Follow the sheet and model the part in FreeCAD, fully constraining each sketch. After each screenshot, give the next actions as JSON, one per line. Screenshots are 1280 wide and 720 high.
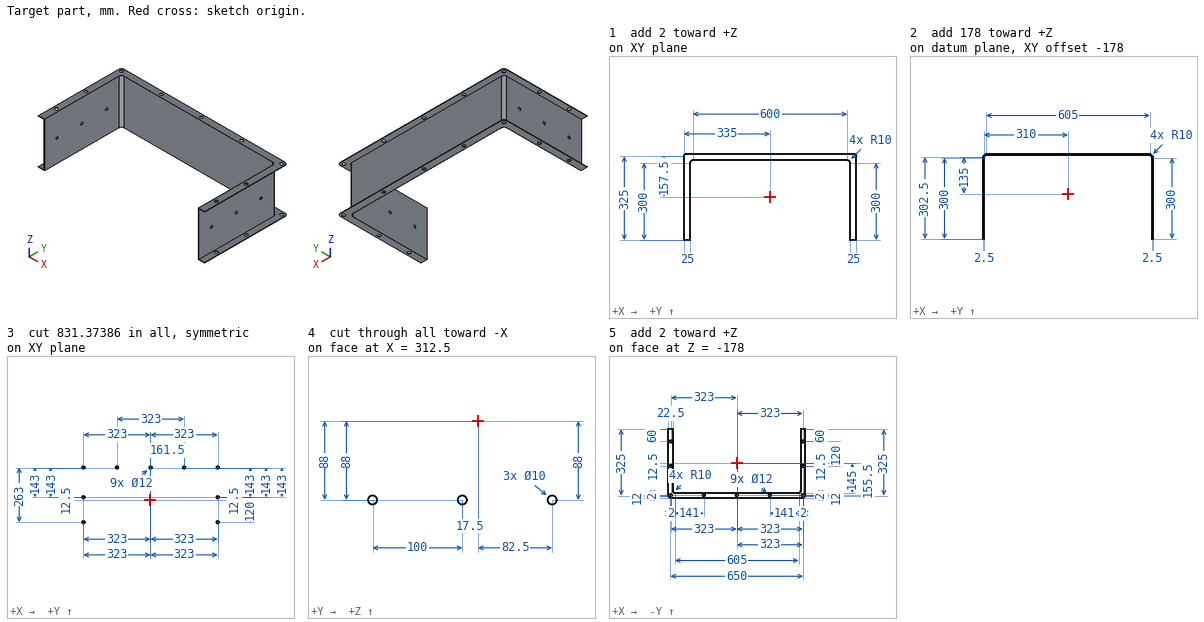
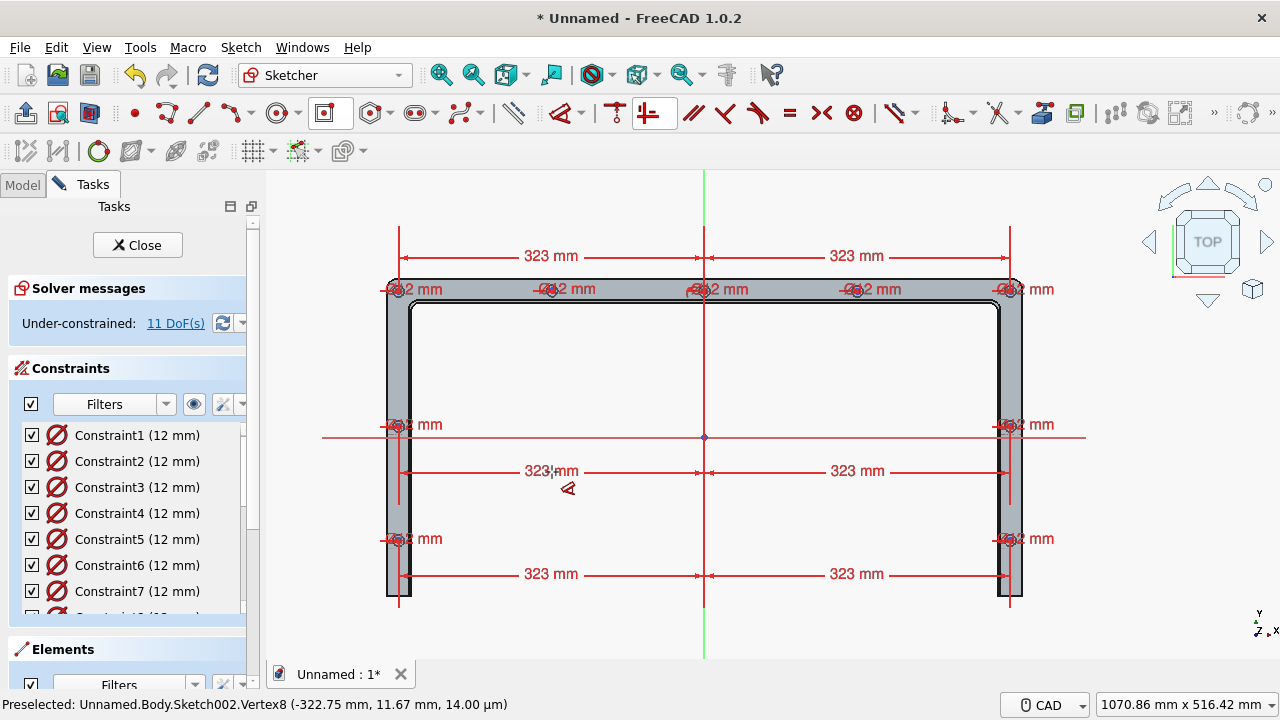
{"action": "scroll", "coordinate": [1010, 427], "scroll_direction": "up", "scroll_amount": 7}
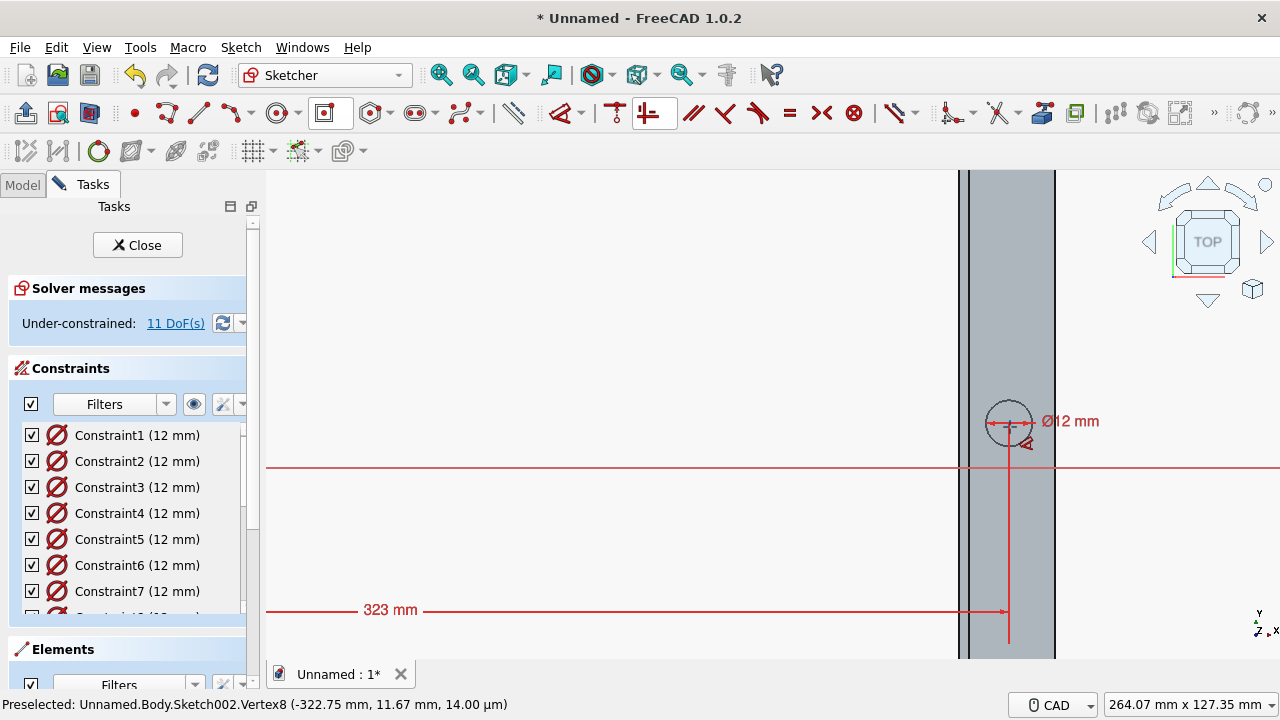
{"action": "left_click", "coordinate": [1009, 423]}
{"action": "left_click", "coordinate": [1043, 446]}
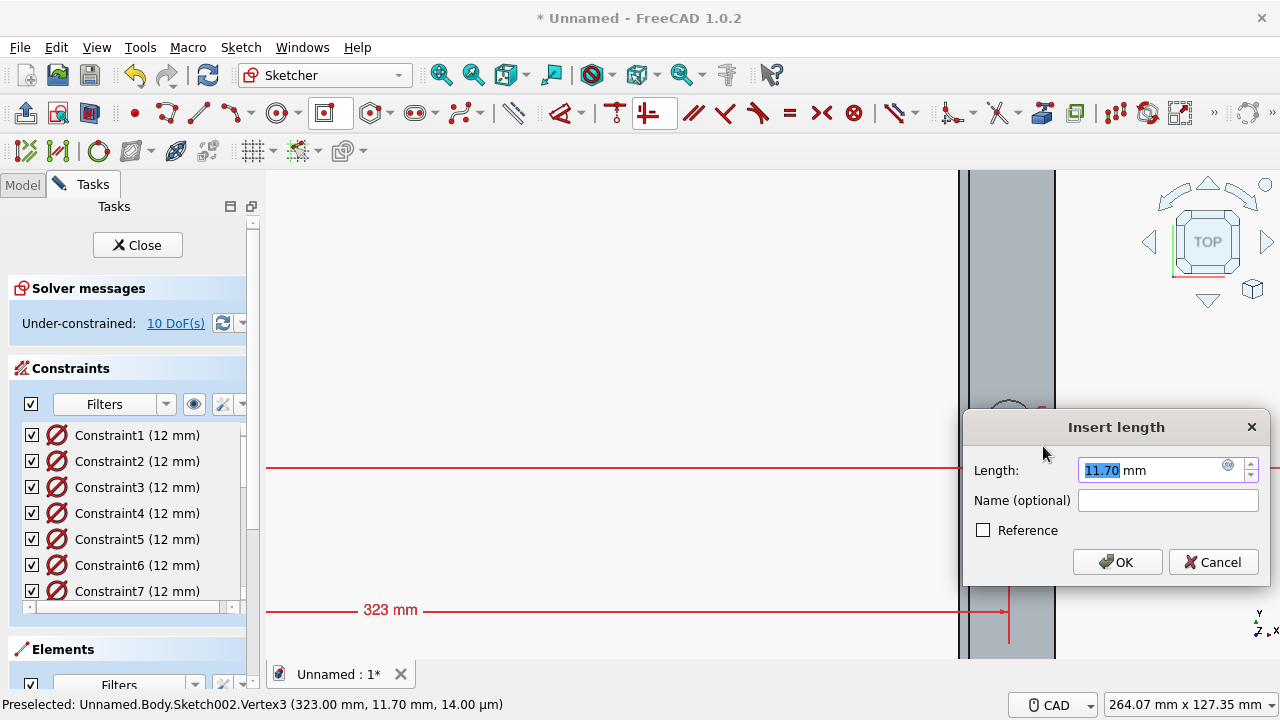
{"action": "type", "text": "12.5"}
{"action": "key", "text": "Return"}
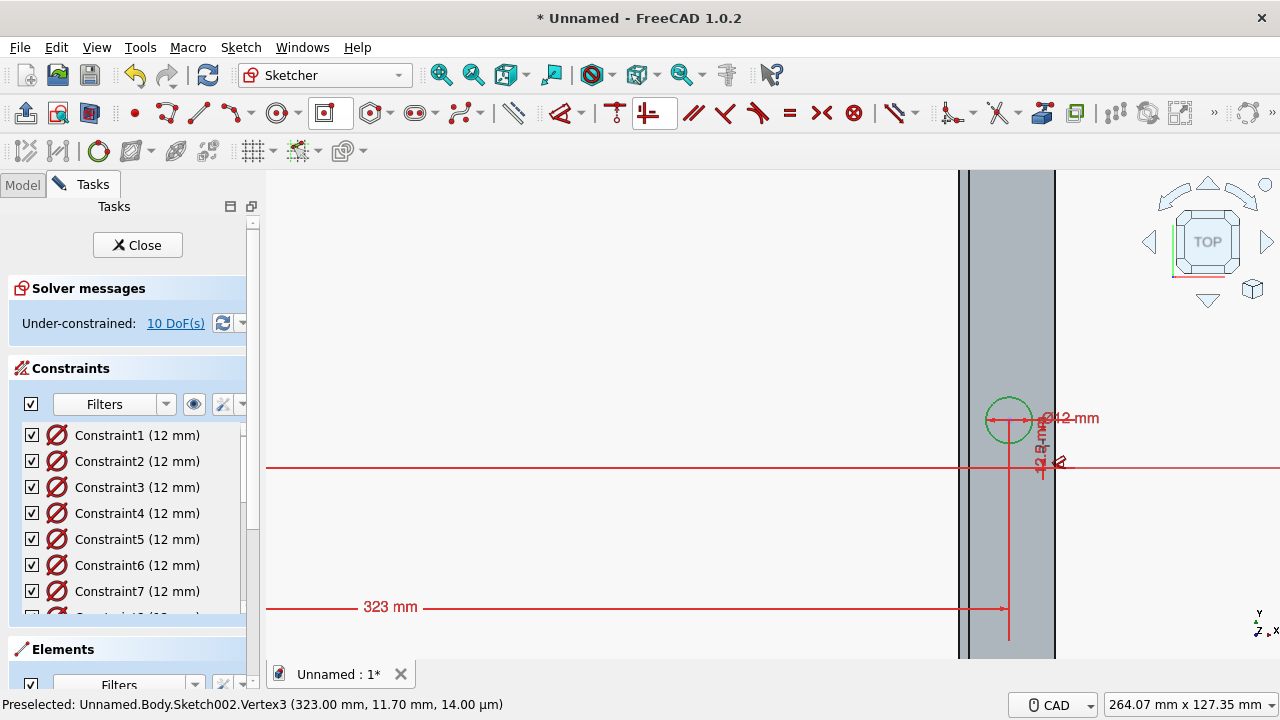
{"action": "scroll", "coordinate": [1011, 427], "scroll_direction": "down", "scroll_amount": 7}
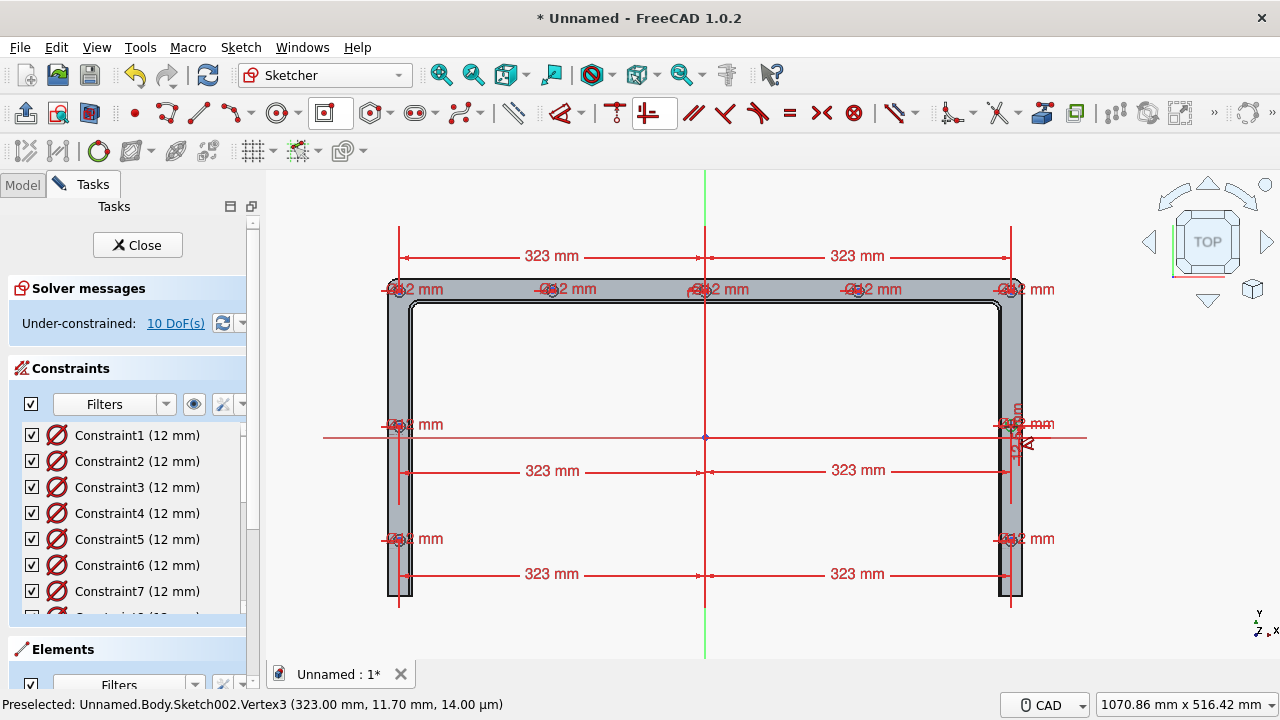
{"action": "scroll", "coordinate": [399, 427], "scroll_direction": "up", "scroll_amount": 7}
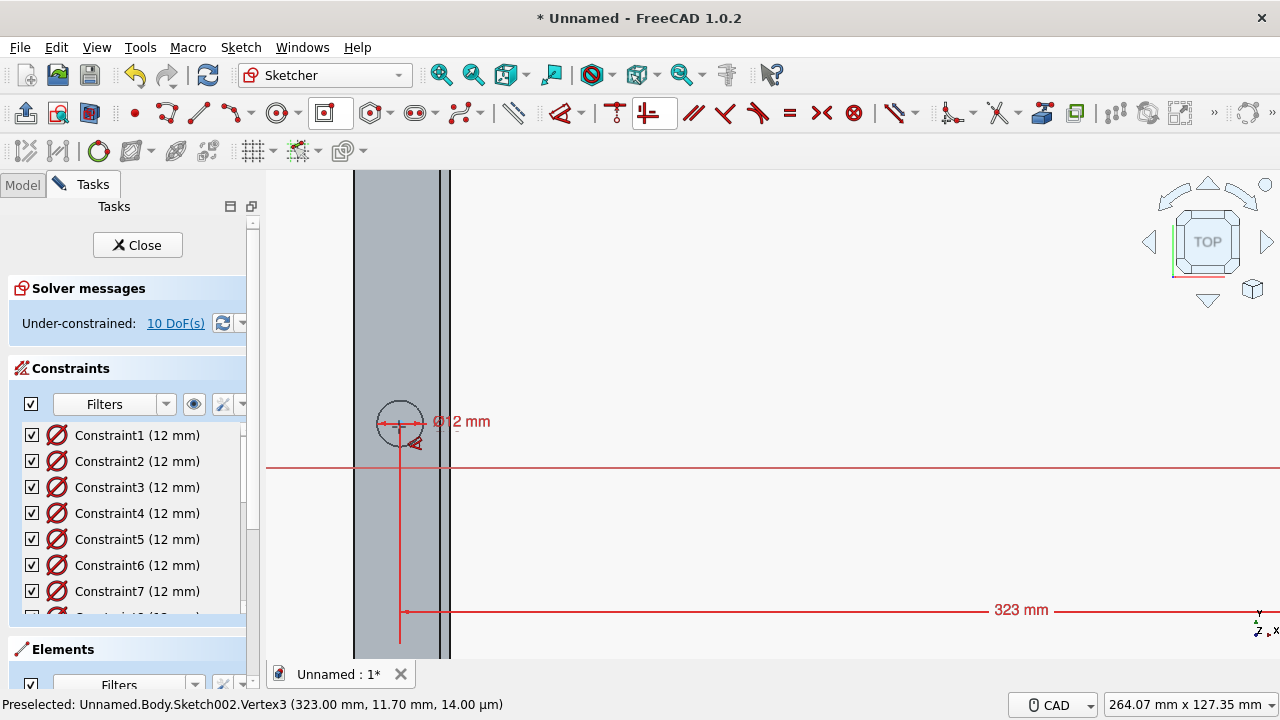
{"action": "left_click", "coordinate": [400, 424]}
{"action": "left_click", "coordinate": [366, 446]}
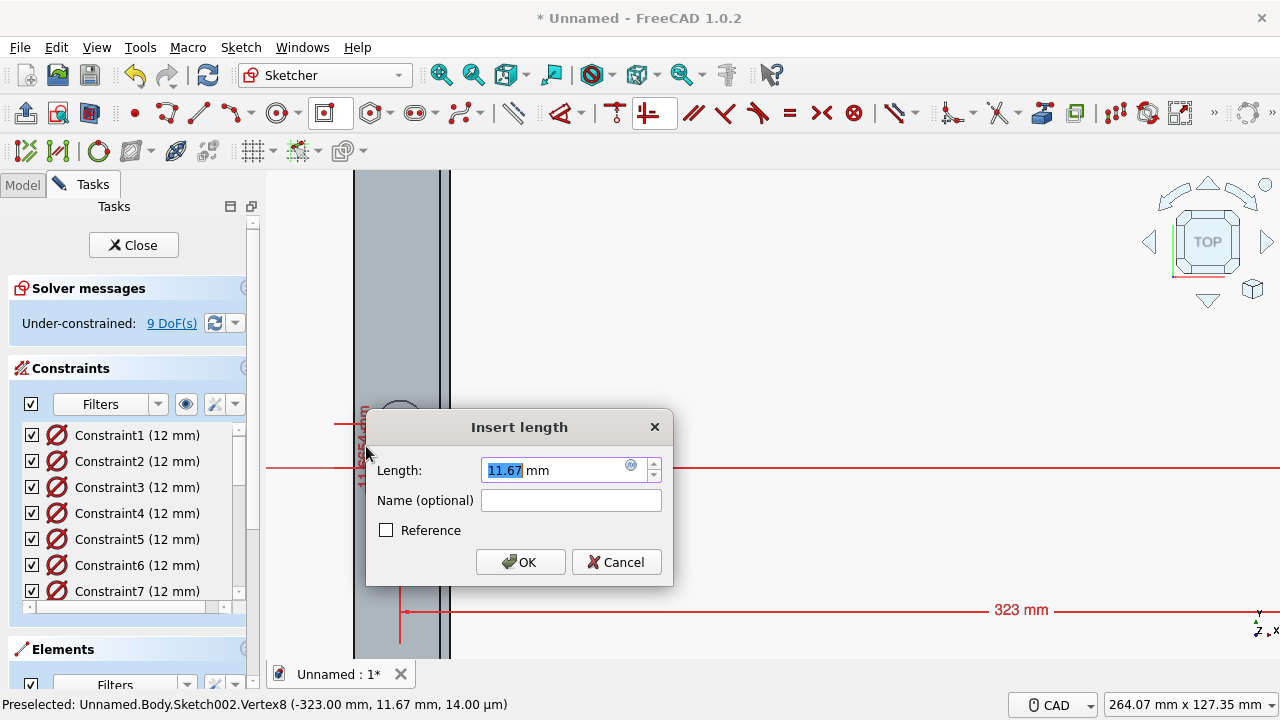
{"action": "type", "text": "12.5"}
{"action": "key", "text": "Return"}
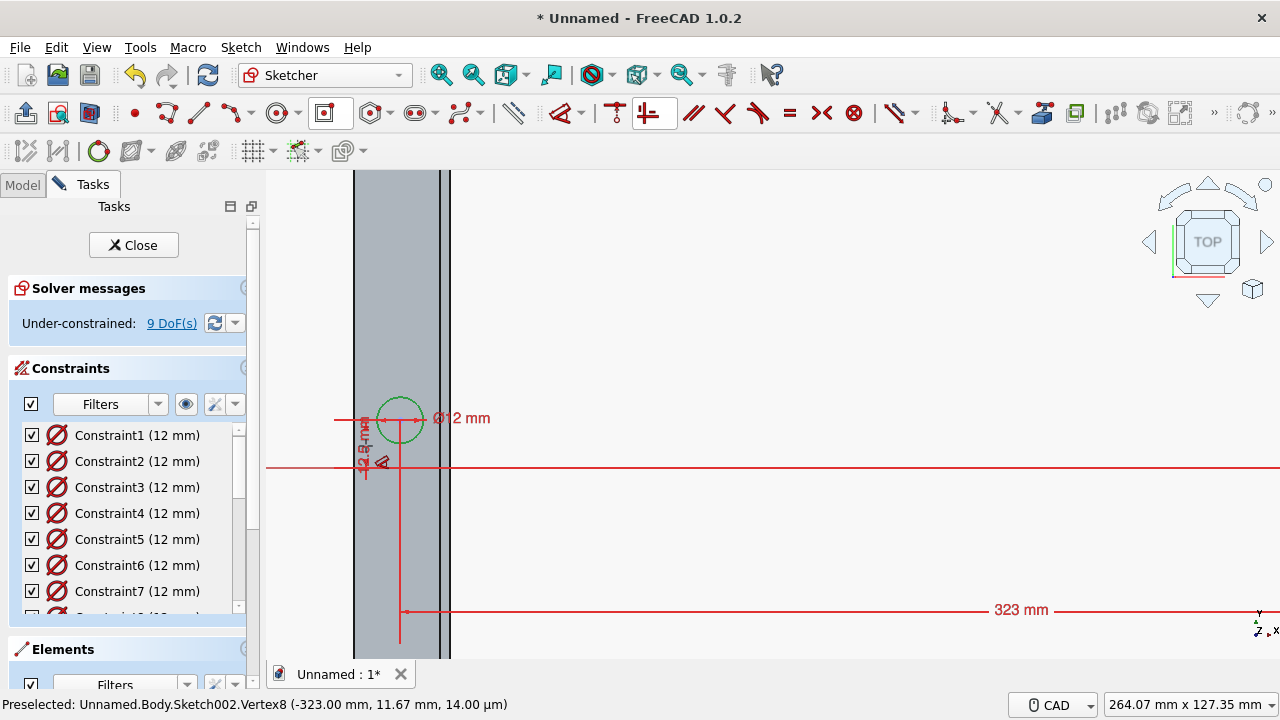
{"action": "scroll", "coordinate": [398, 427], "scroll_direction": "down", "scroll_amount": 7}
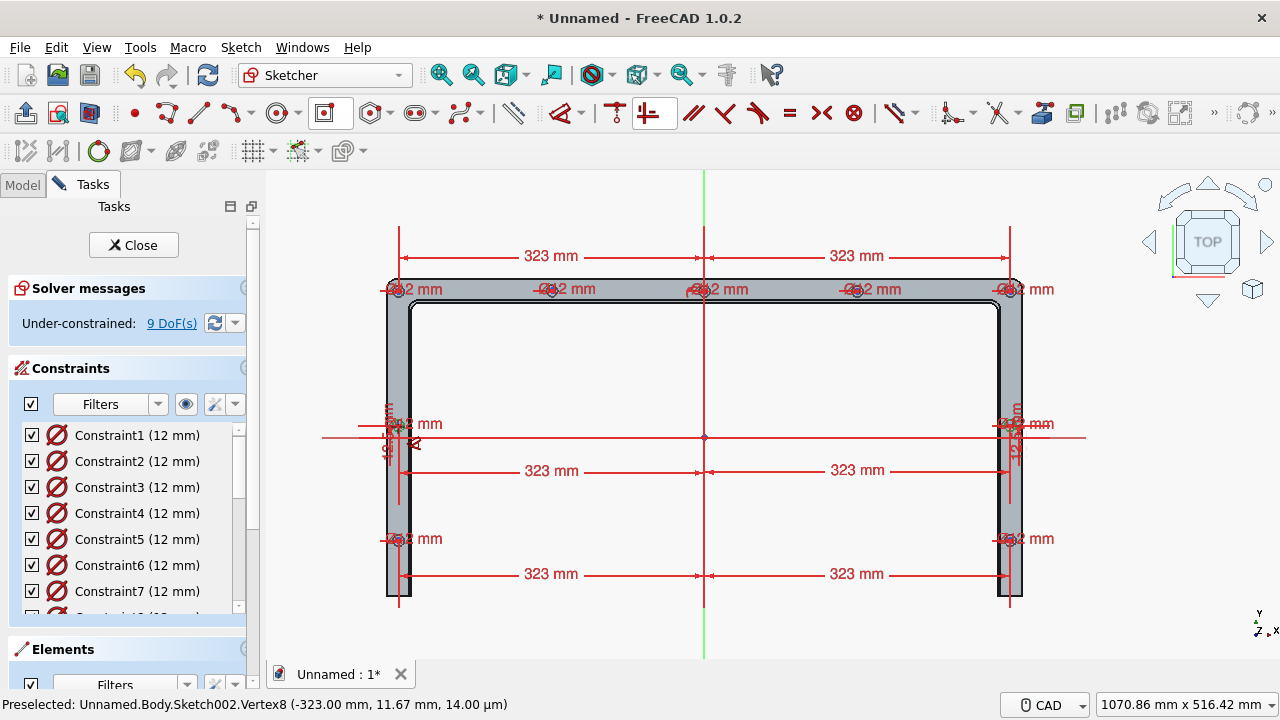
{"action": "left_click", "coordinate": [857, 291]}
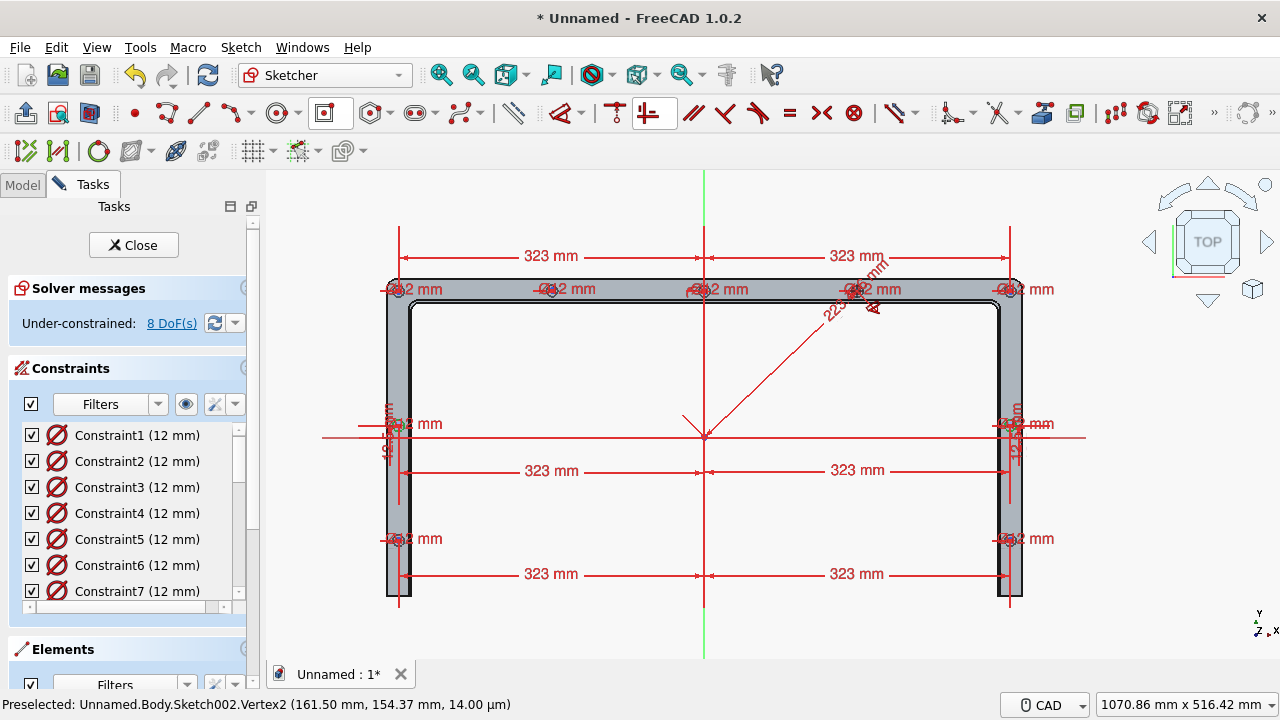
{"action": "left_click", "coordinate": [1010, 426]}
{"action": "left_click", "coordinate": [1044, 359]}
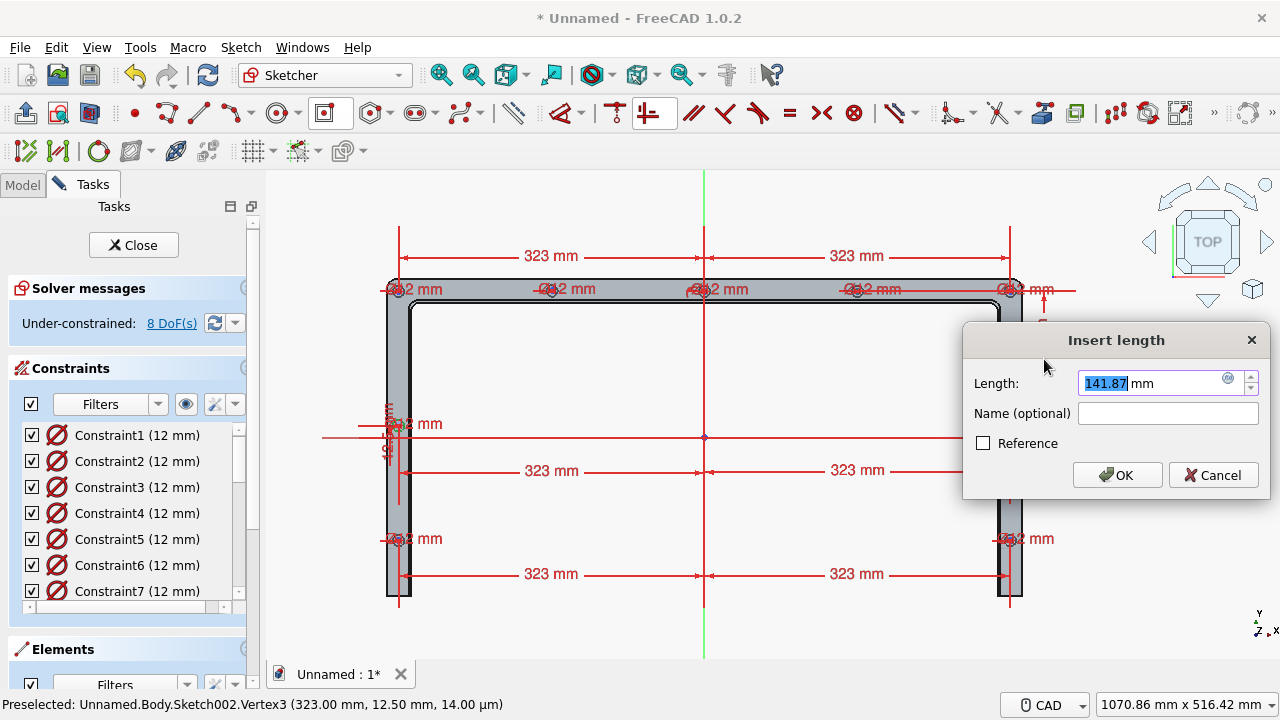
{"action": "type", "text": "143"}
{"action": "key", "text": "Return"}